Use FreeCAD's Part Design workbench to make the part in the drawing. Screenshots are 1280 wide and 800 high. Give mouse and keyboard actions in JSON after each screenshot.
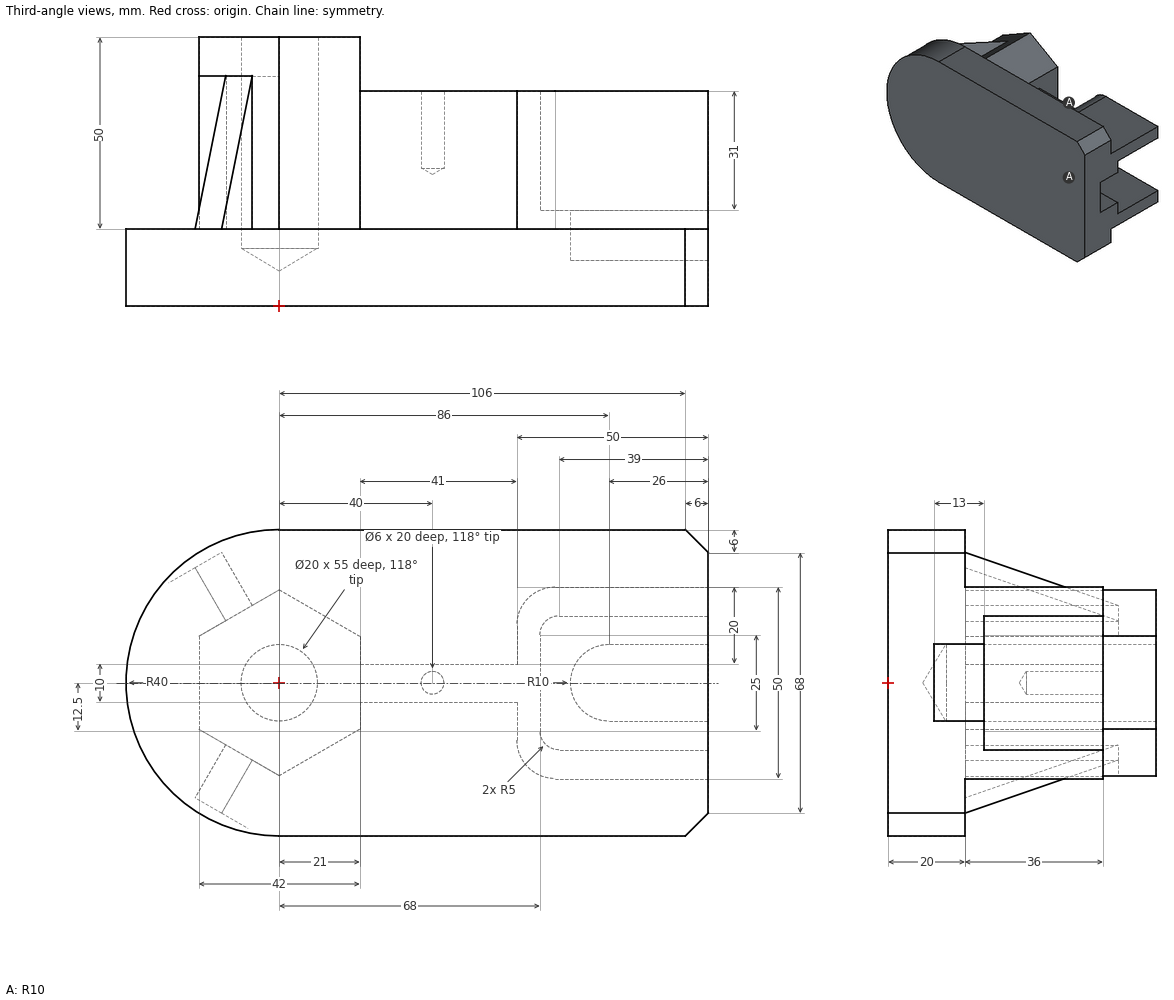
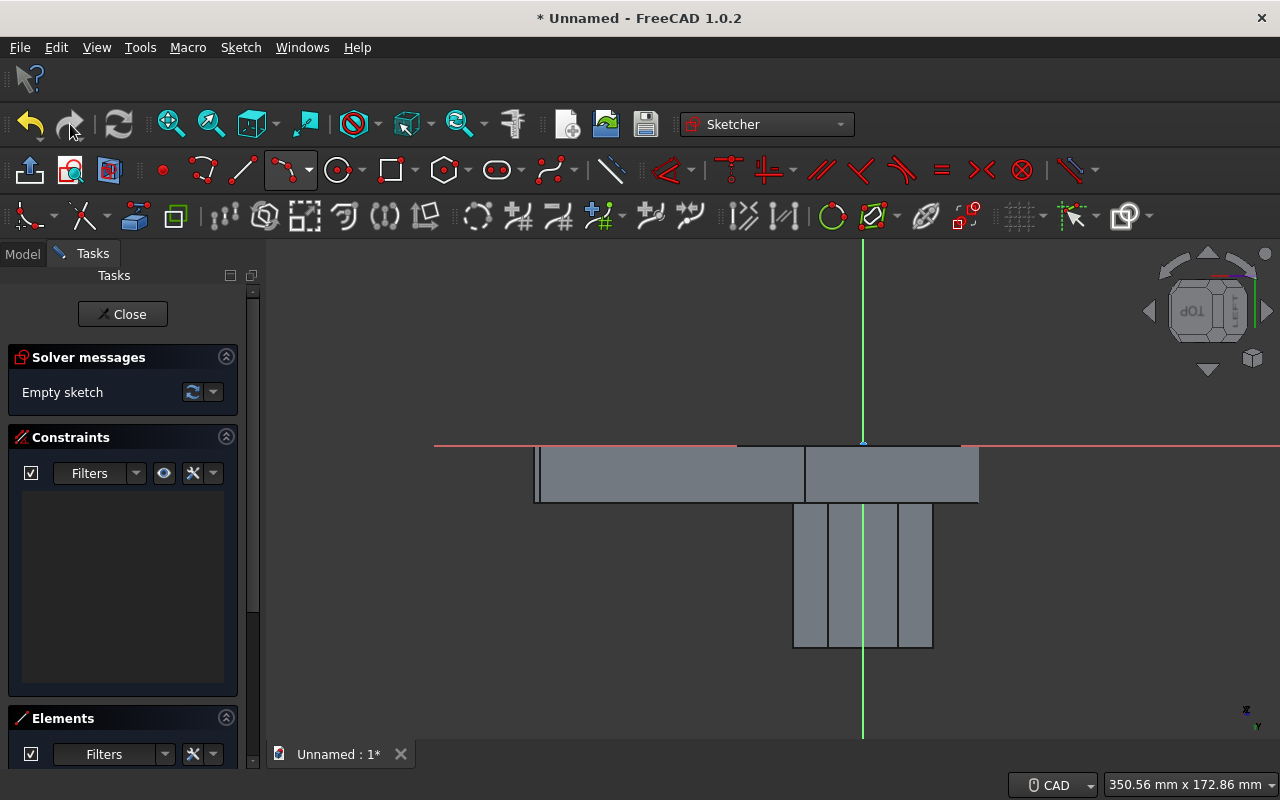
{"action": "scroll", "coordinate": [1056, 585], "scroll_direction": "up", "scroll_amount": 3}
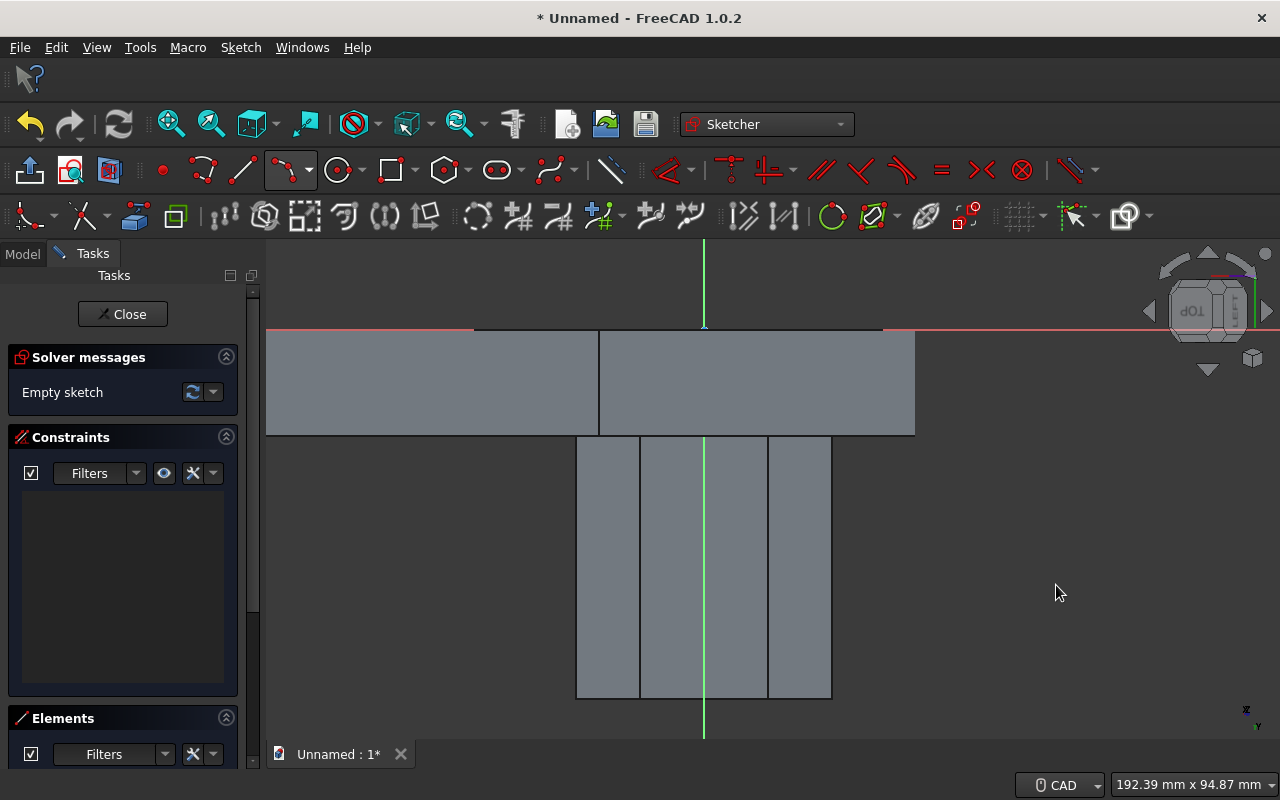
{"action": "left_click", "coordinate": [392, 170]}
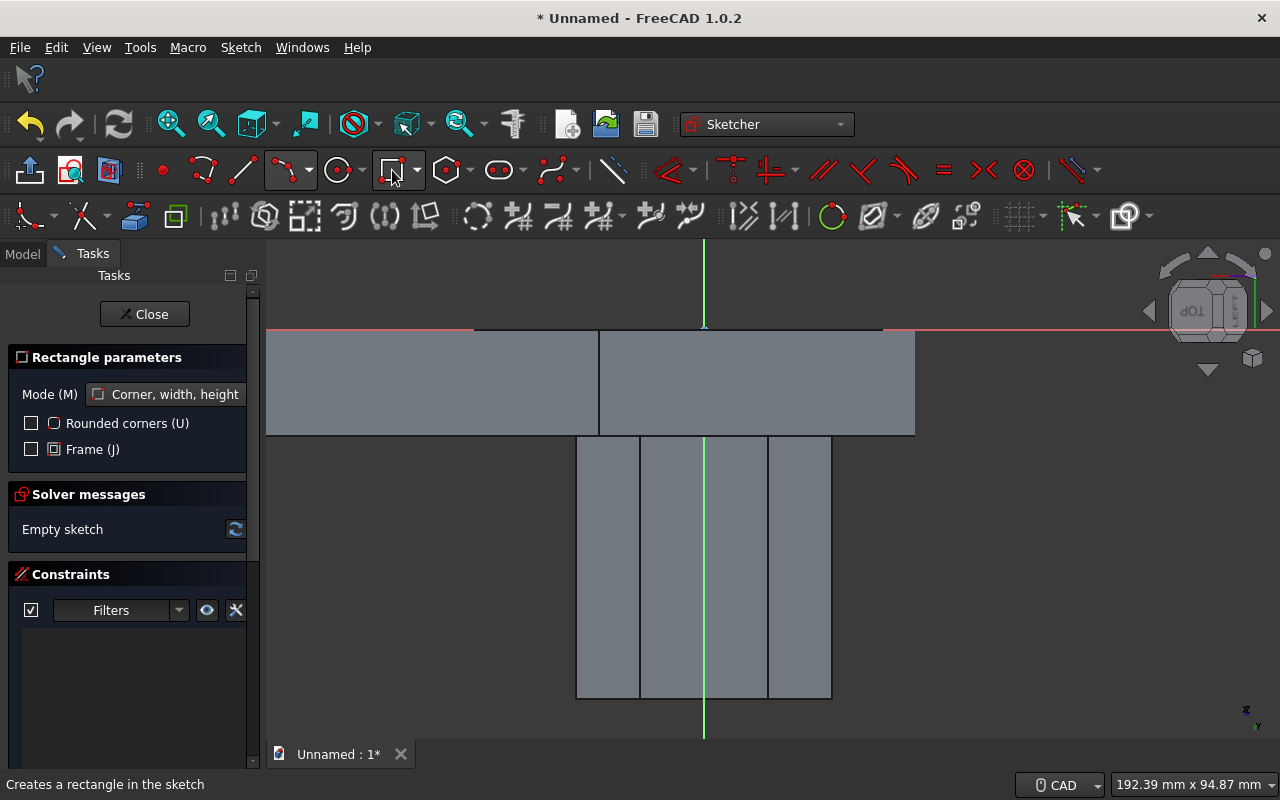
{"action": "left_click", "coordinate": [683, 436]}
{"action": "mouse_move", "coordinate": [725, 647]}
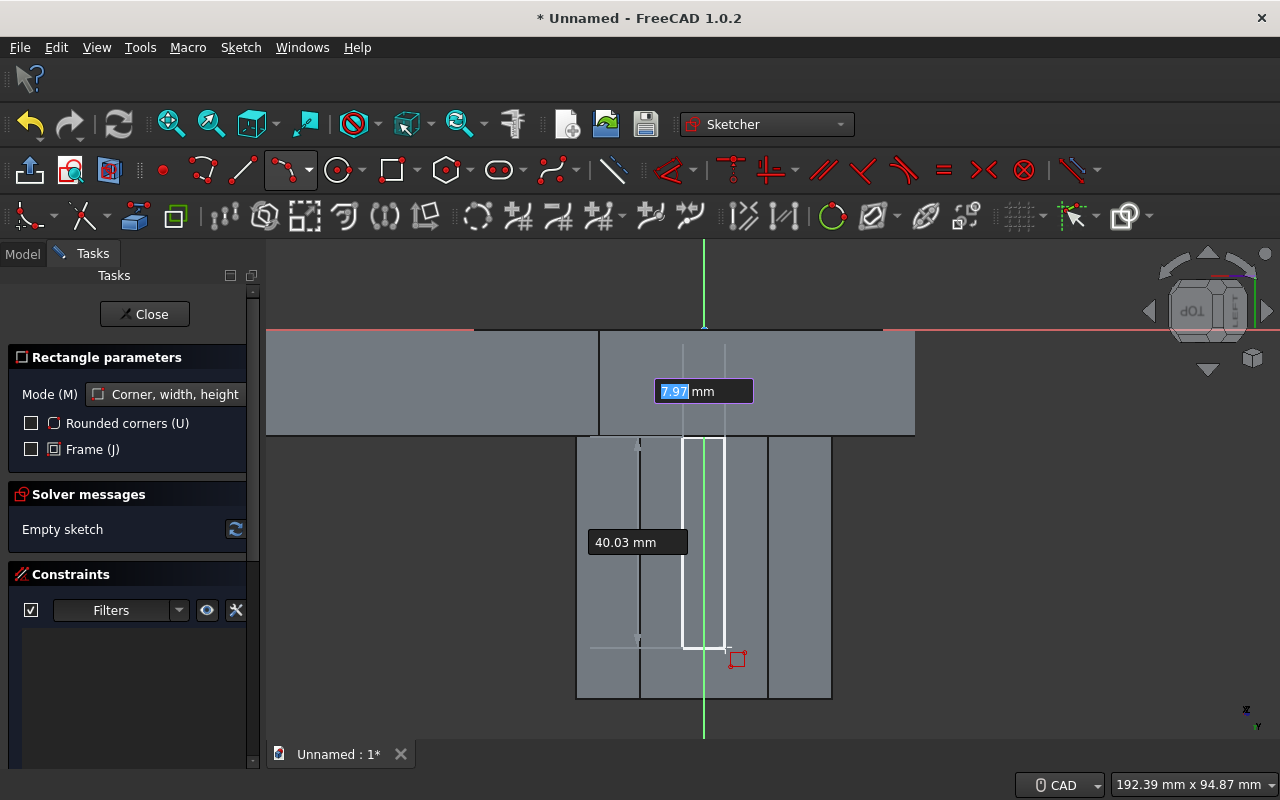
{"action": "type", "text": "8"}
{"action": "key", "text": "Tab"}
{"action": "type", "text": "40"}
{"action": "key", "text": "Return"}
{"action": "key", "text": "Escape"}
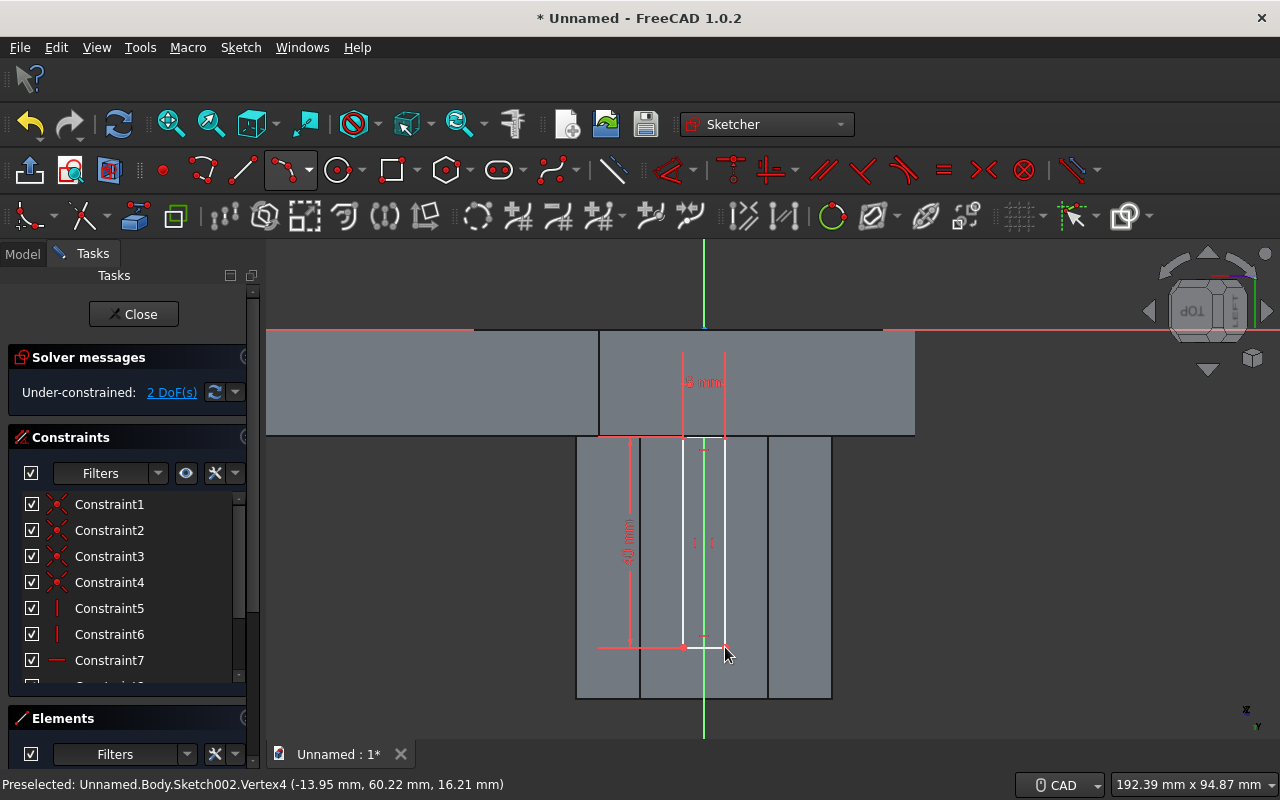
{"action": "left_click", "coordinate": [668, 170]}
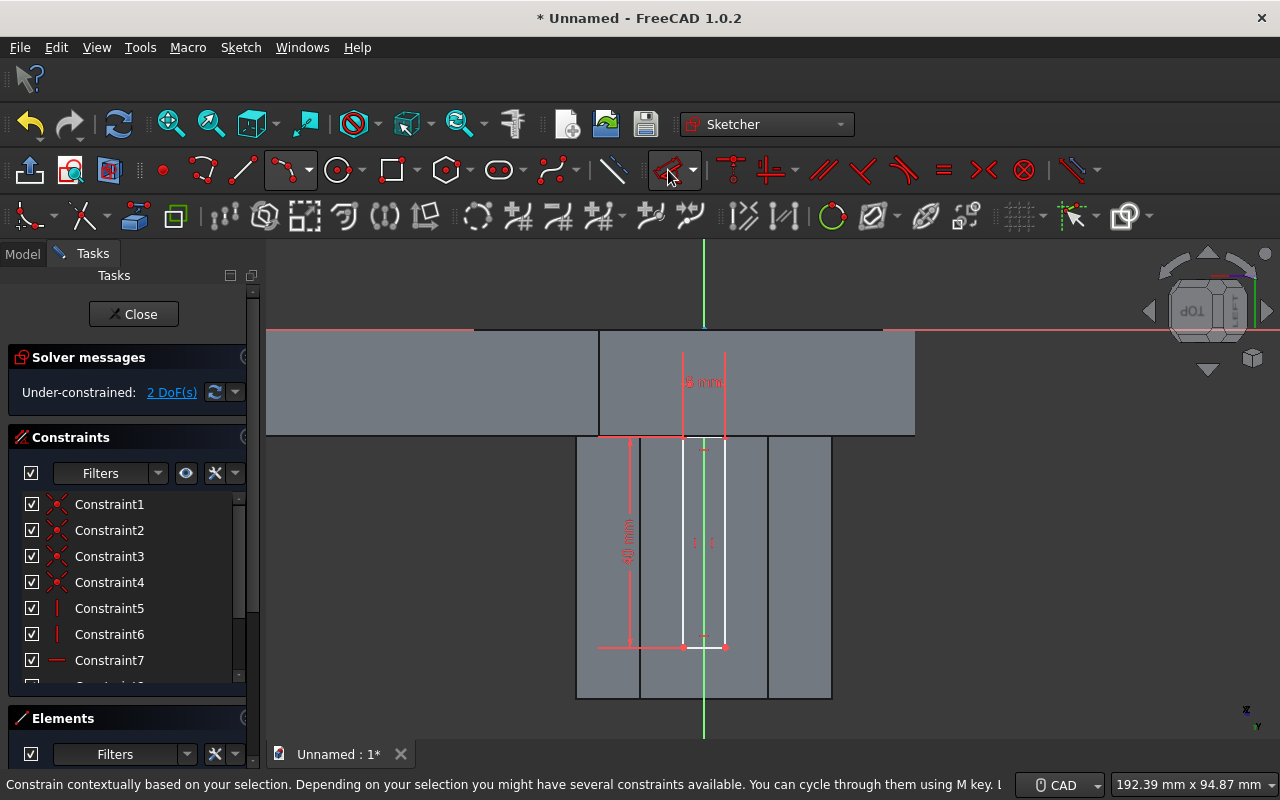
{"action": "scroll", "coordinate": [683, 437], "scroll_direction": "up", "scroll_amount": 4}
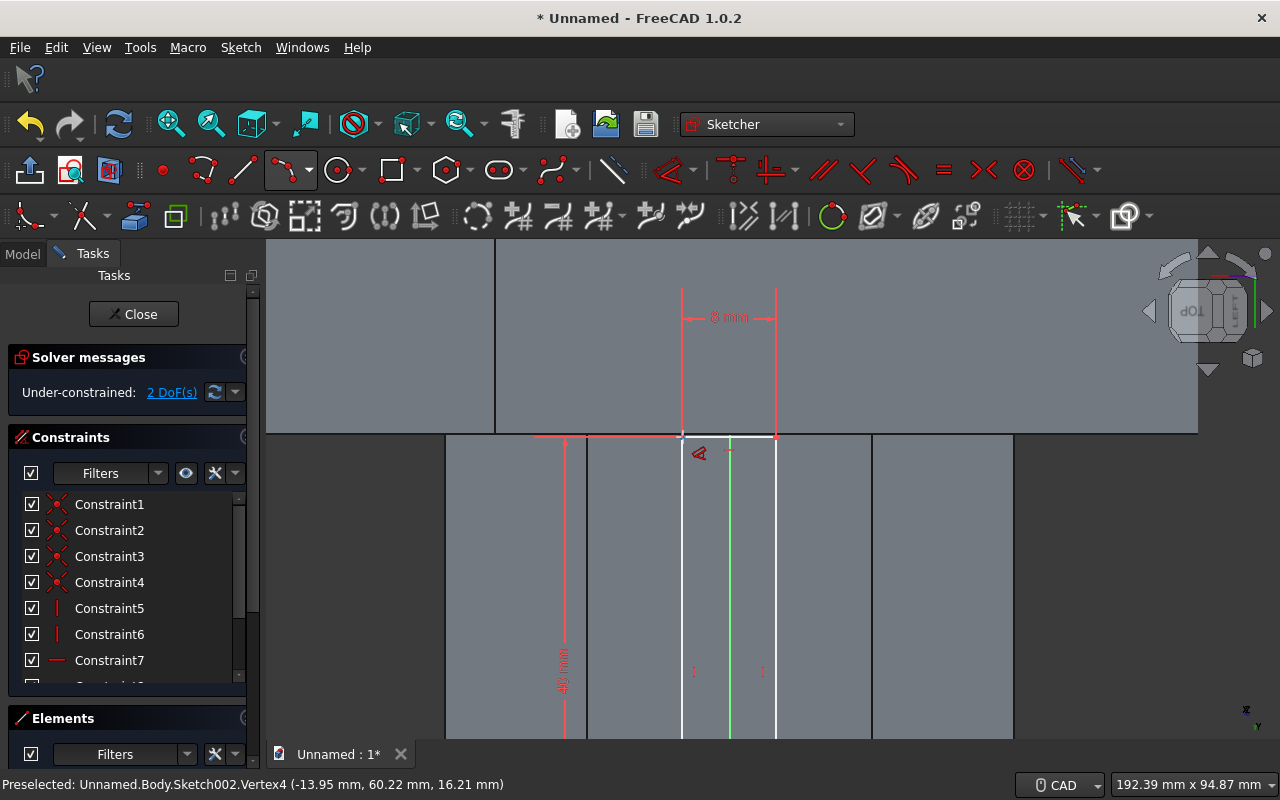
{"action": "left_click", "coordinate": [682, 437]}
{"action": "left_click", "coordinate": [706, 471]}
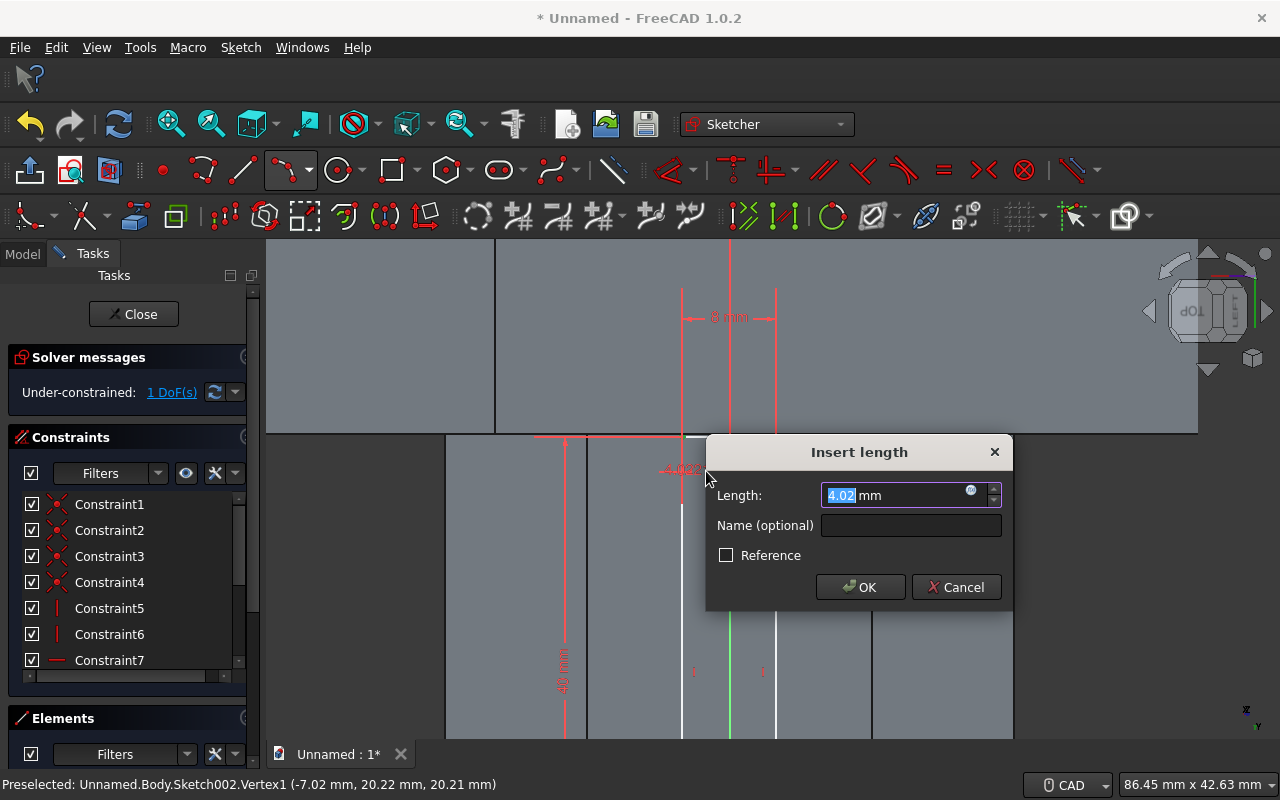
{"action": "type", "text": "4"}
{"action": "key", "text": "Return"}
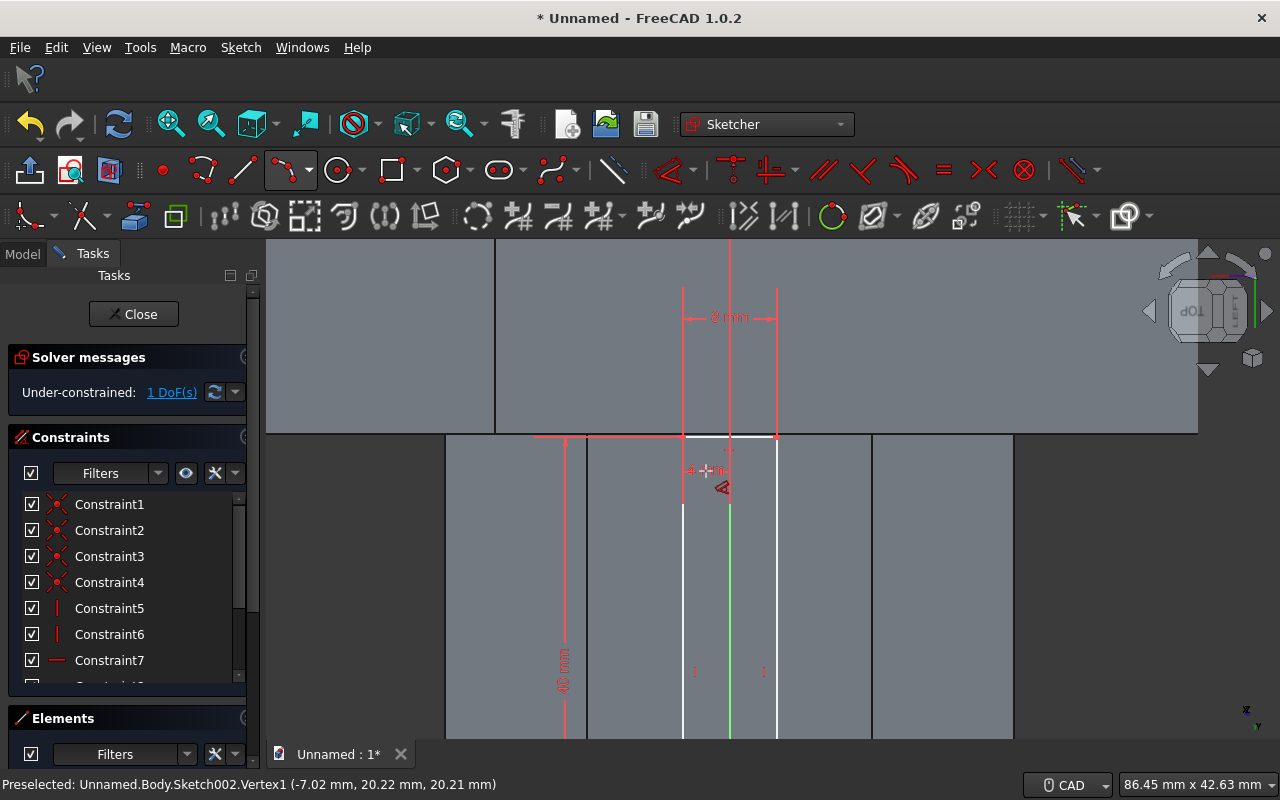
{"action": "left_click", "coordinate": [683, 437]}
{"action": "left_click", "coordinate": [649, 352]}